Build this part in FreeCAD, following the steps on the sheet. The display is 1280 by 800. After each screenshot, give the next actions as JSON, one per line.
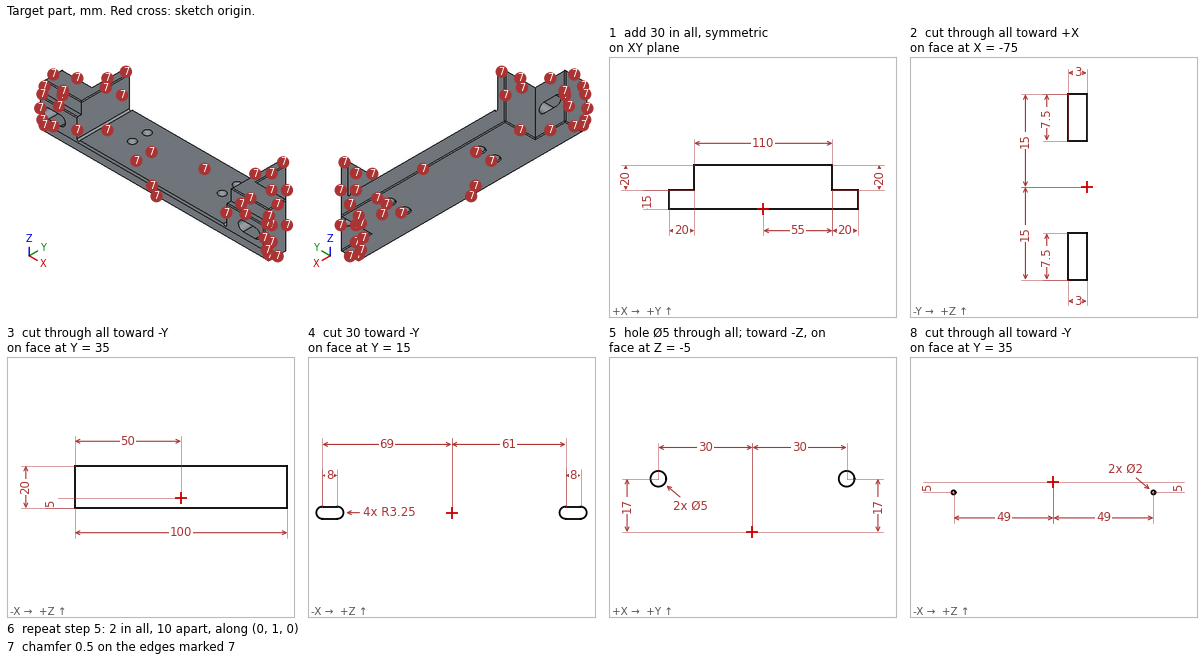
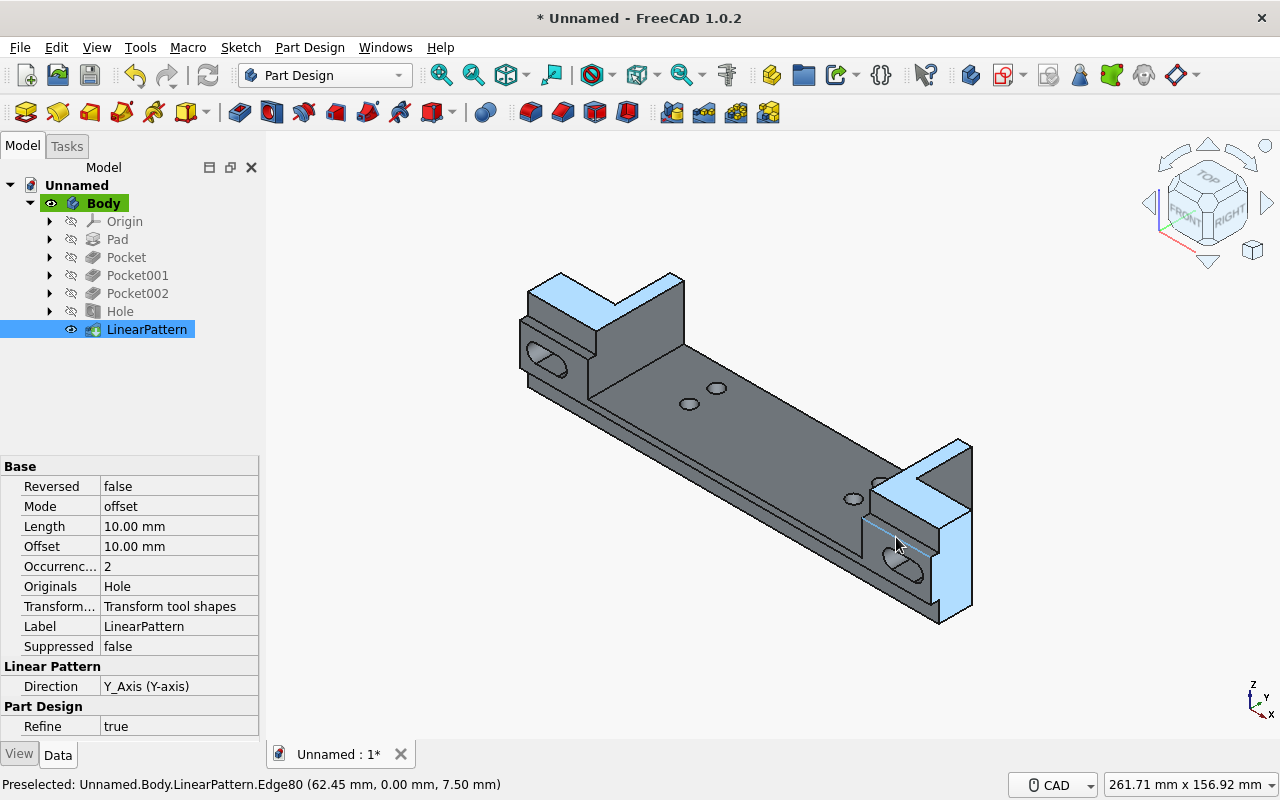
{"action": "left_click", "coordinate": [554, 339], "text": "ctrl"}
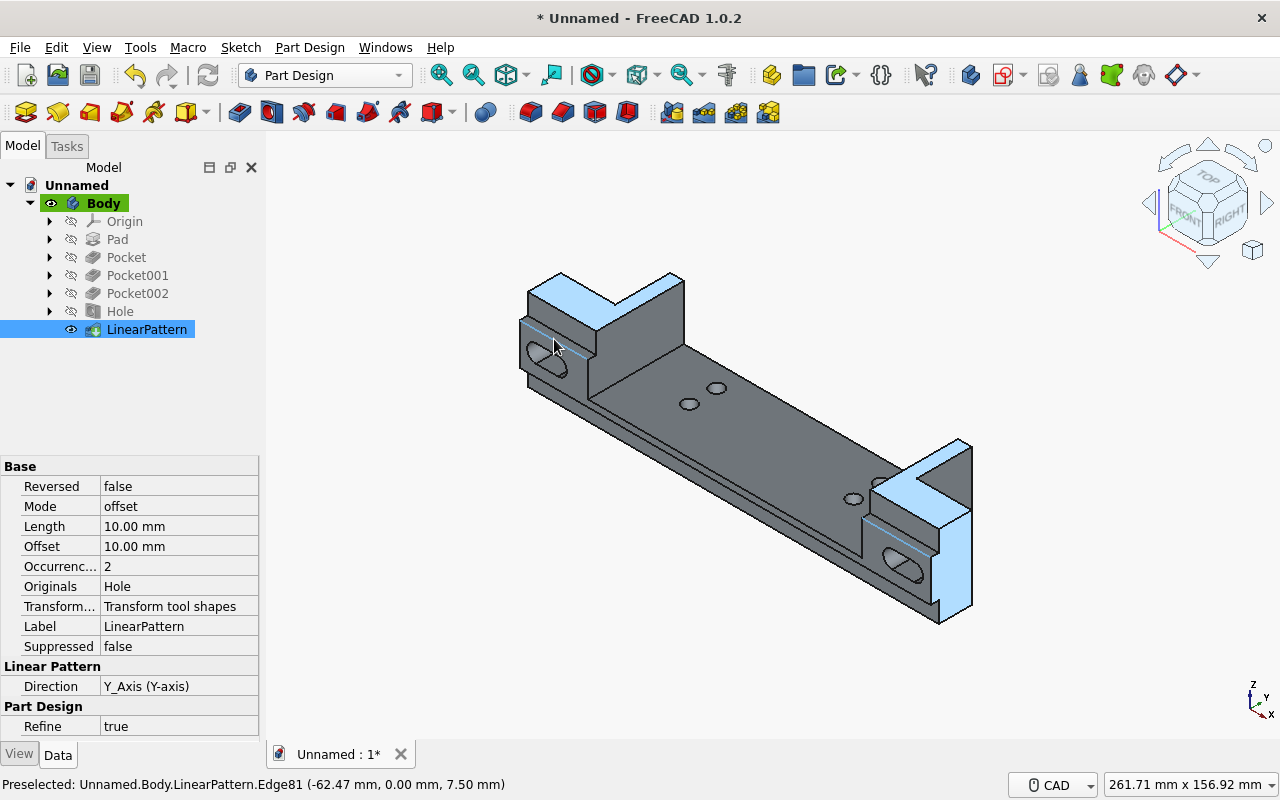
{"action": "key", "text": "2"}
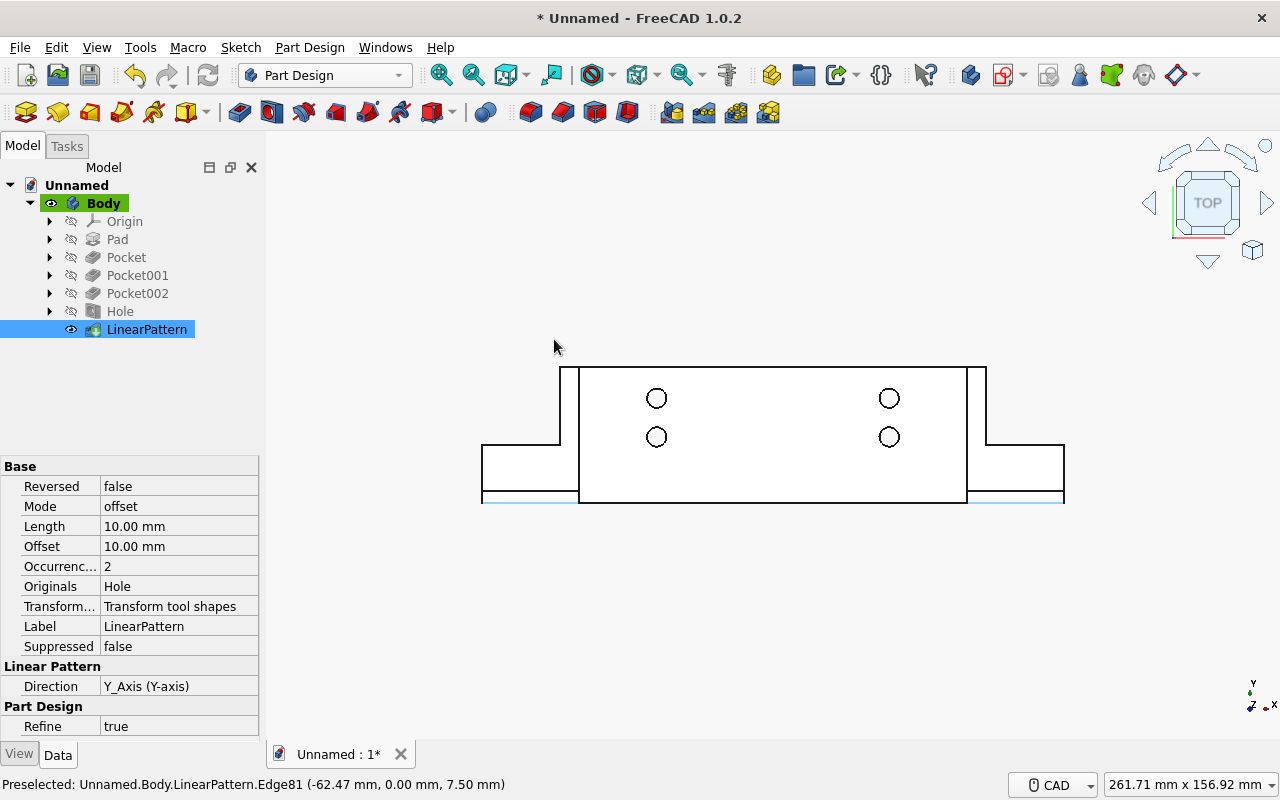
{"action": "key", "text": "0"}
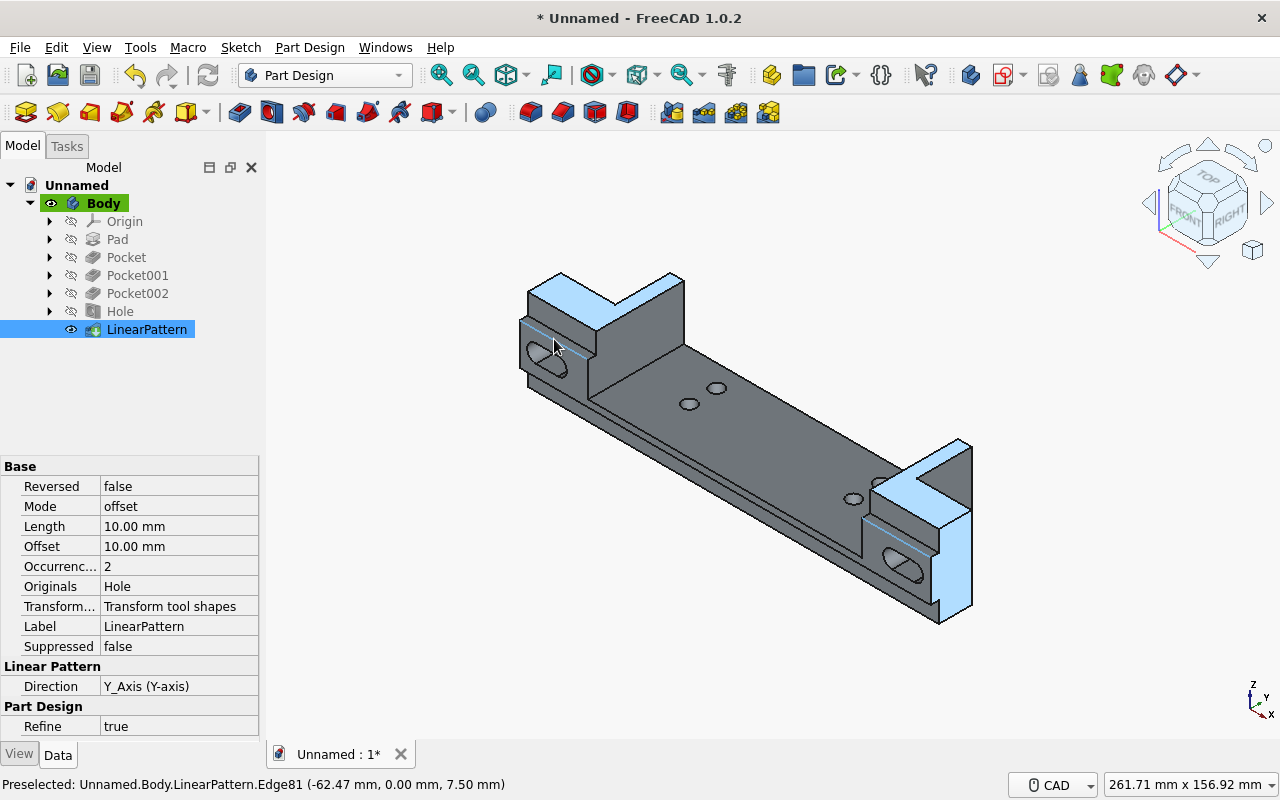
{"action": "key", "text": "1"}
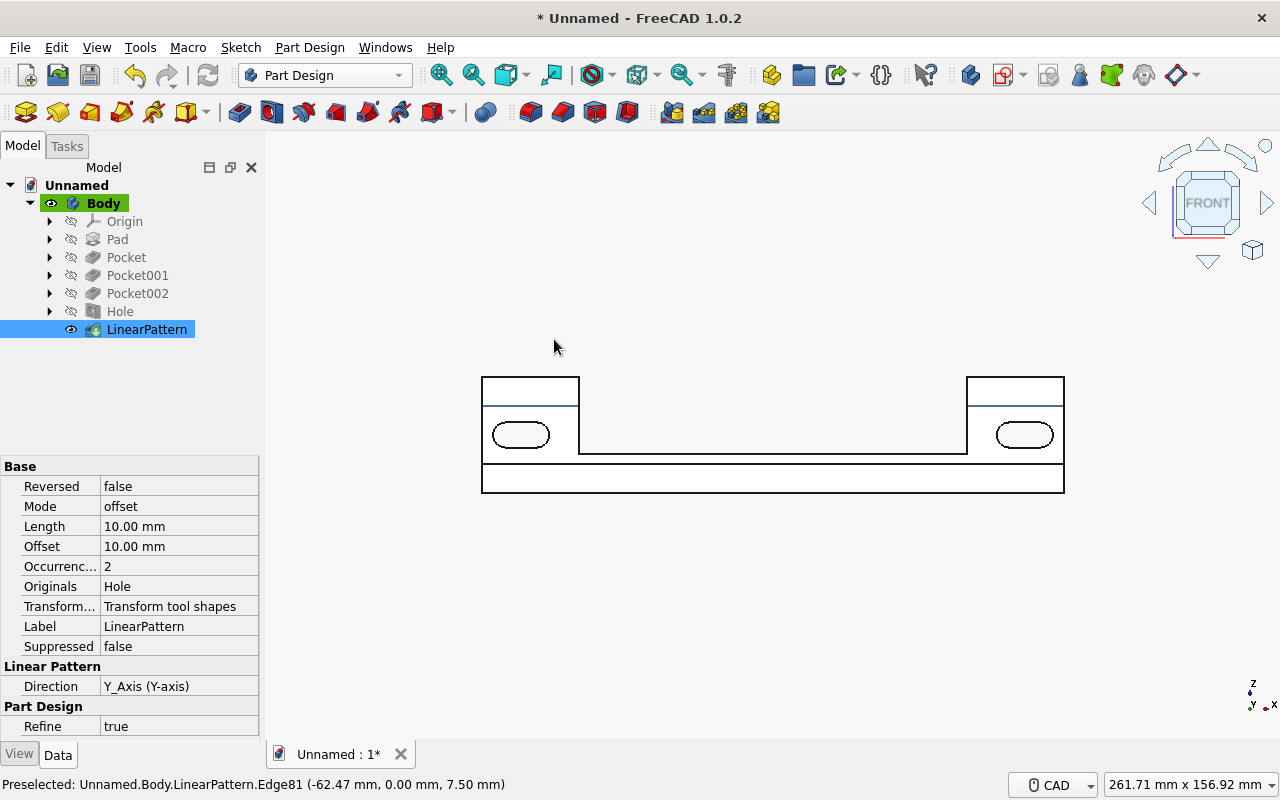
{"action": "left_click", "coordinate": [773, 463], "text": "ctrl"}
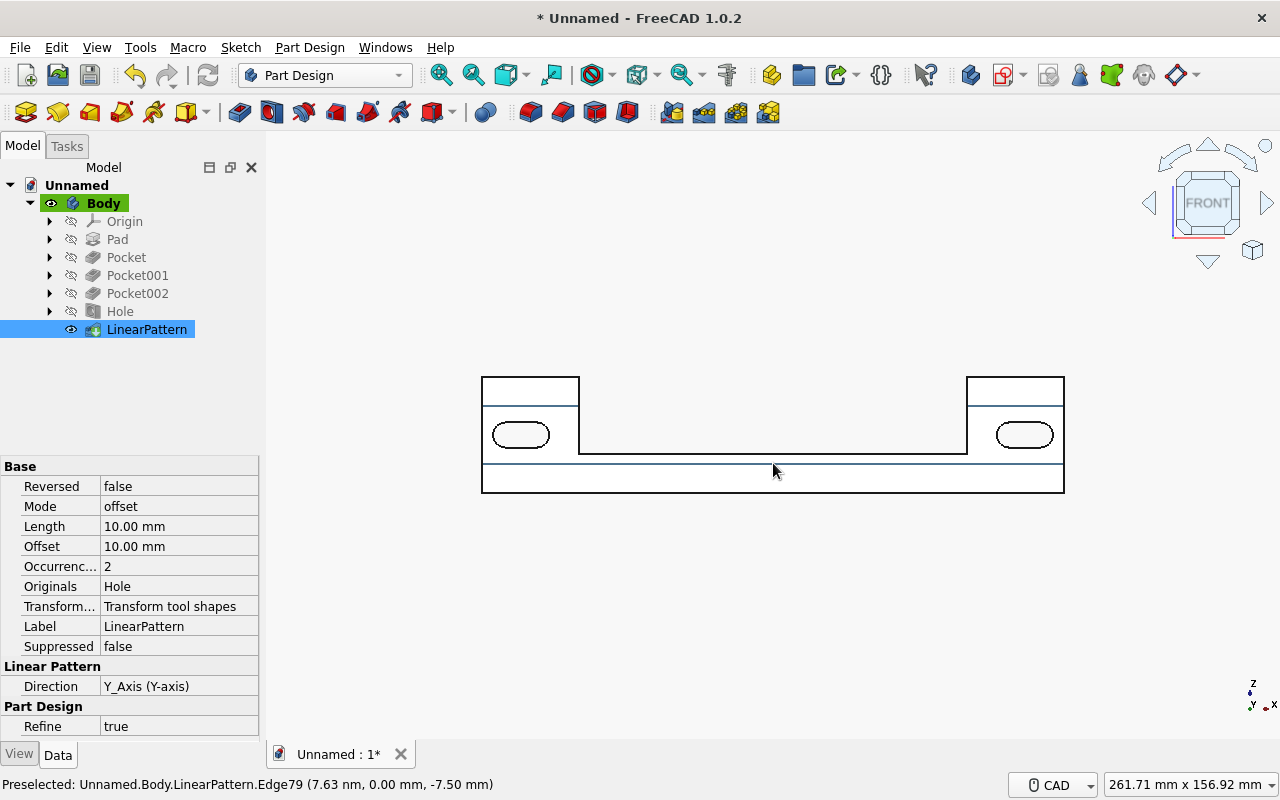
{"action": "key", "text": "3"}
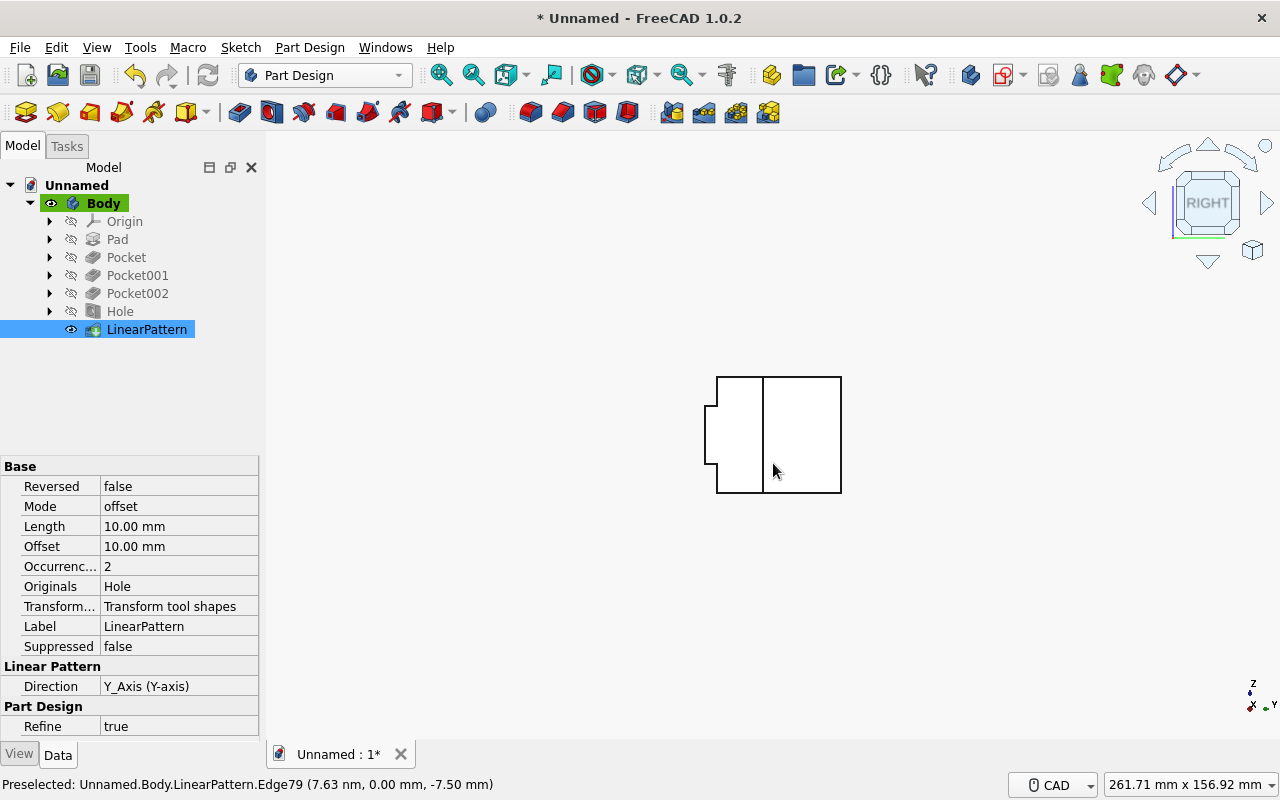
{"action": "key", "text": "v f"}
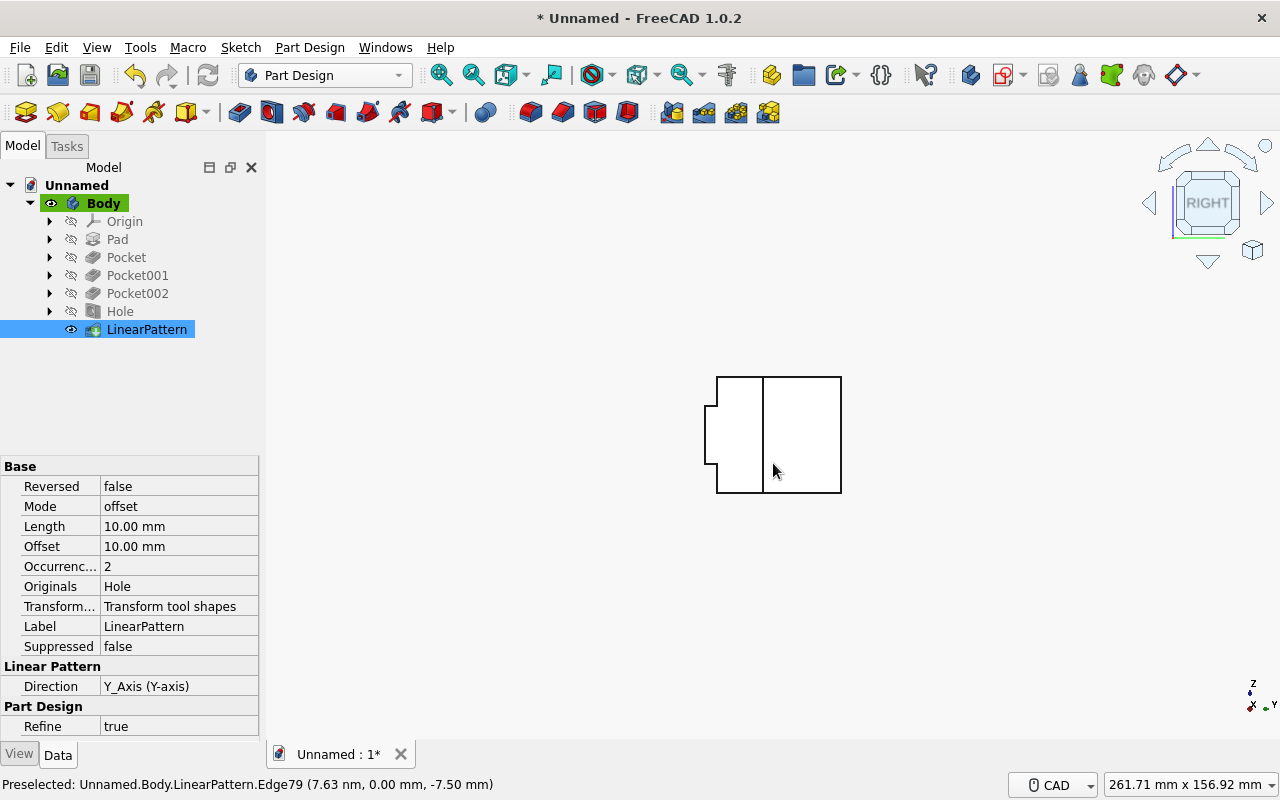
{"action": "left_click", "coordinate": [841, 434], "text": "ctrl"}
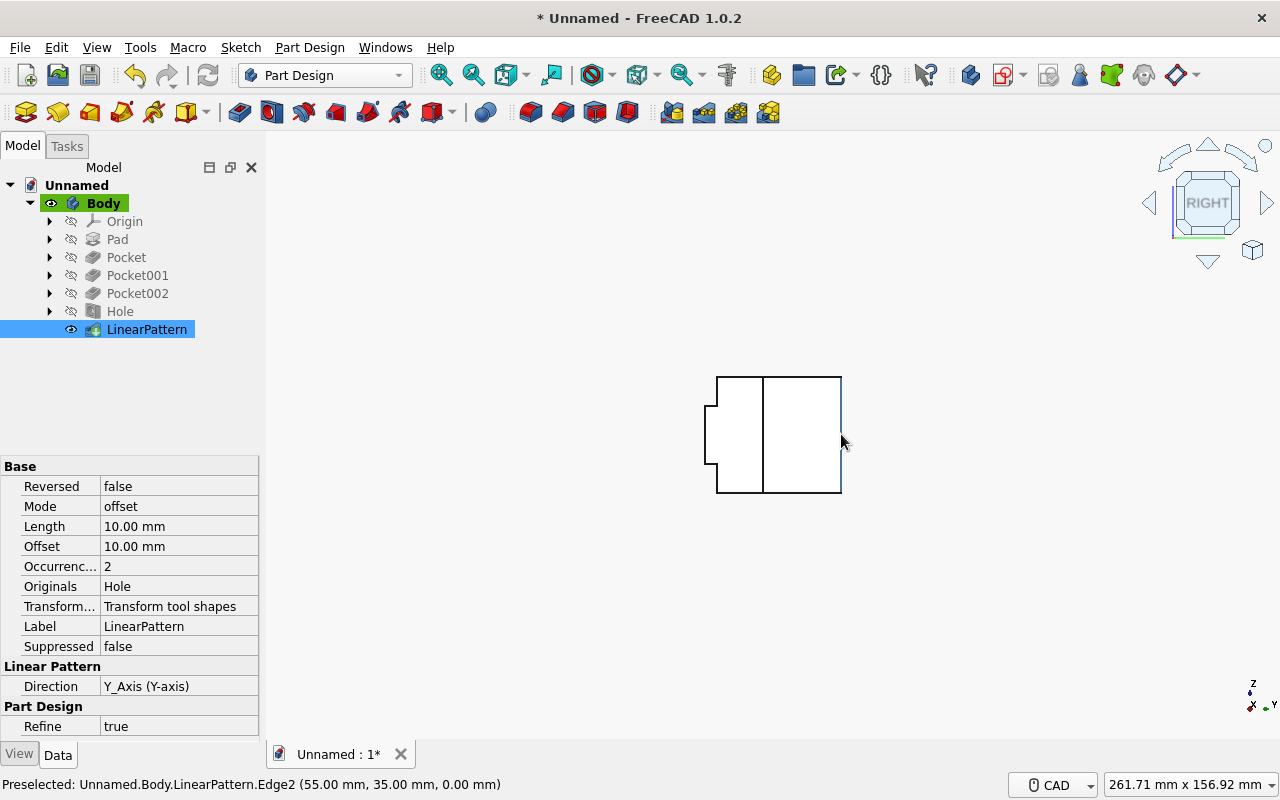
{"action": "key", "text": "5"}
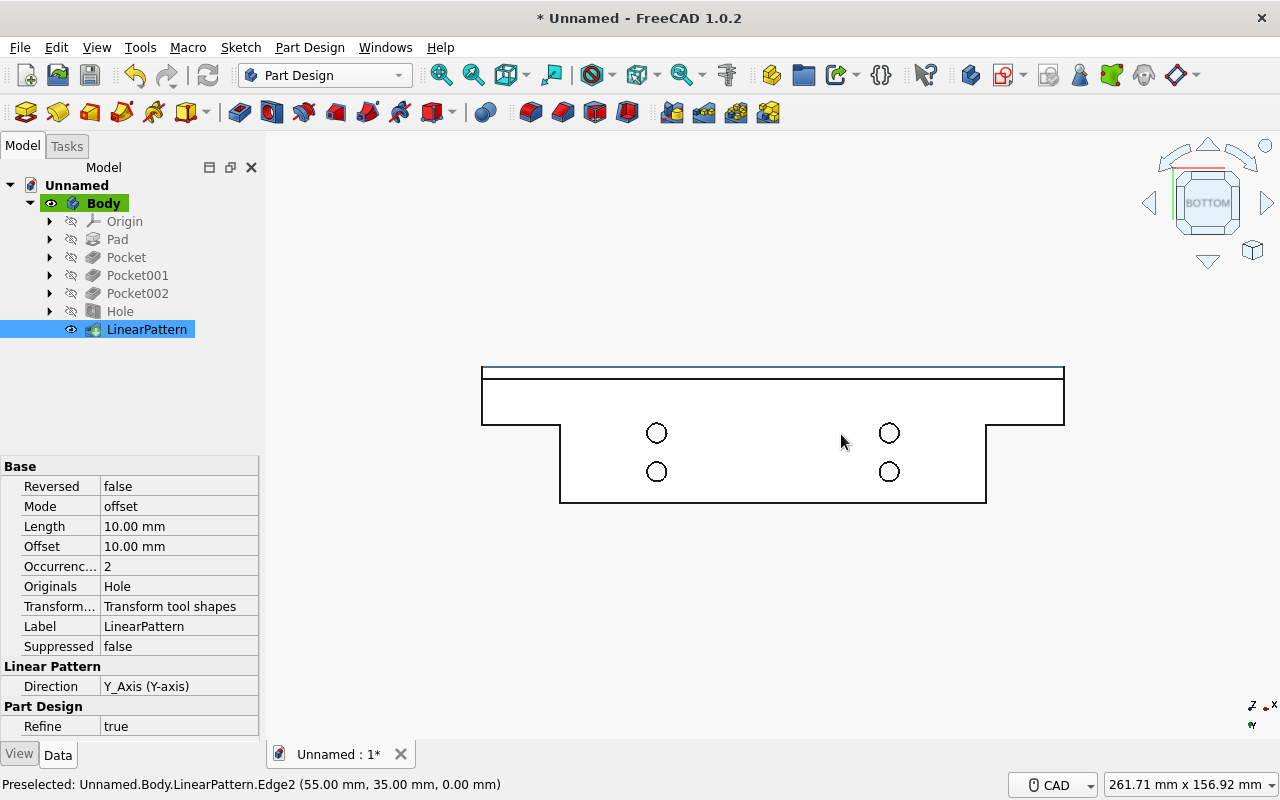
{"action": "left_click", "coordinate": [773, 440], "text": "ctrl"}